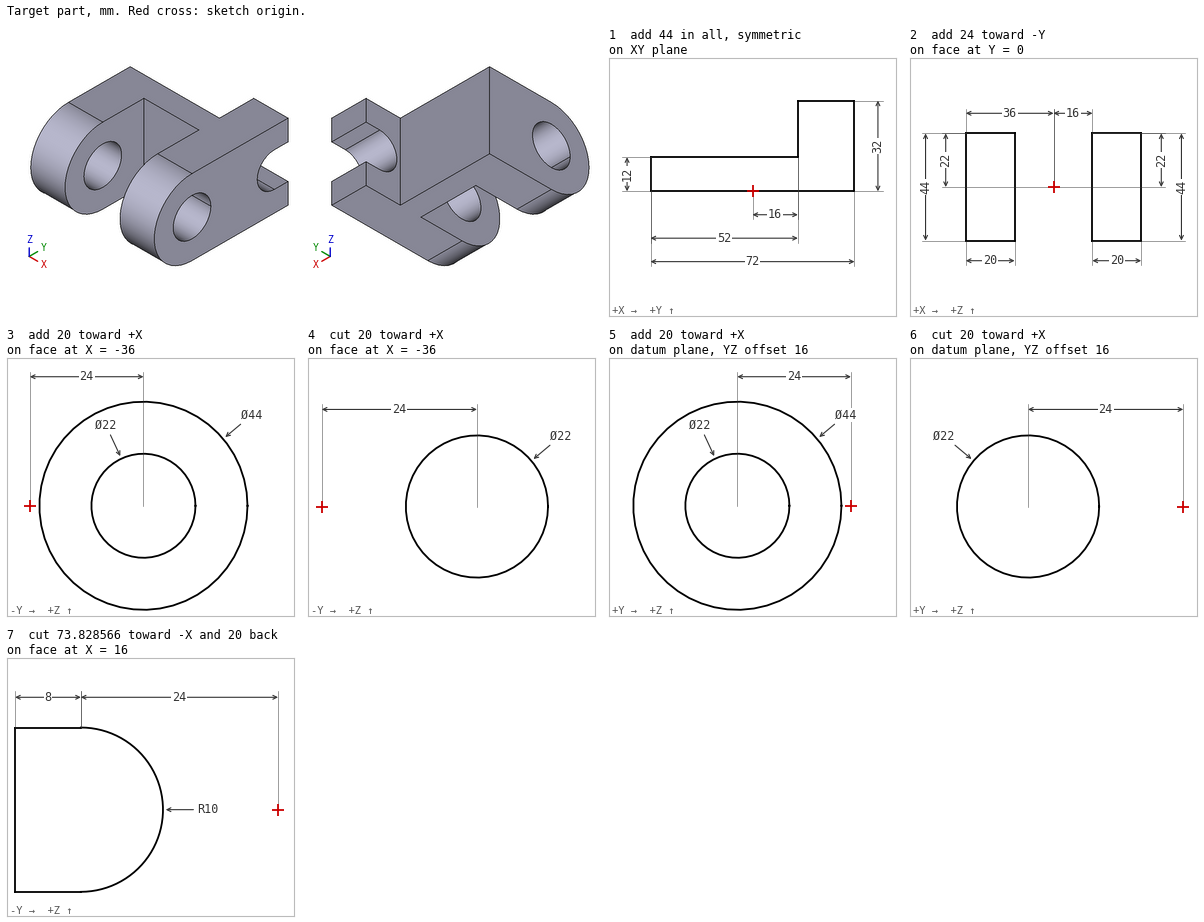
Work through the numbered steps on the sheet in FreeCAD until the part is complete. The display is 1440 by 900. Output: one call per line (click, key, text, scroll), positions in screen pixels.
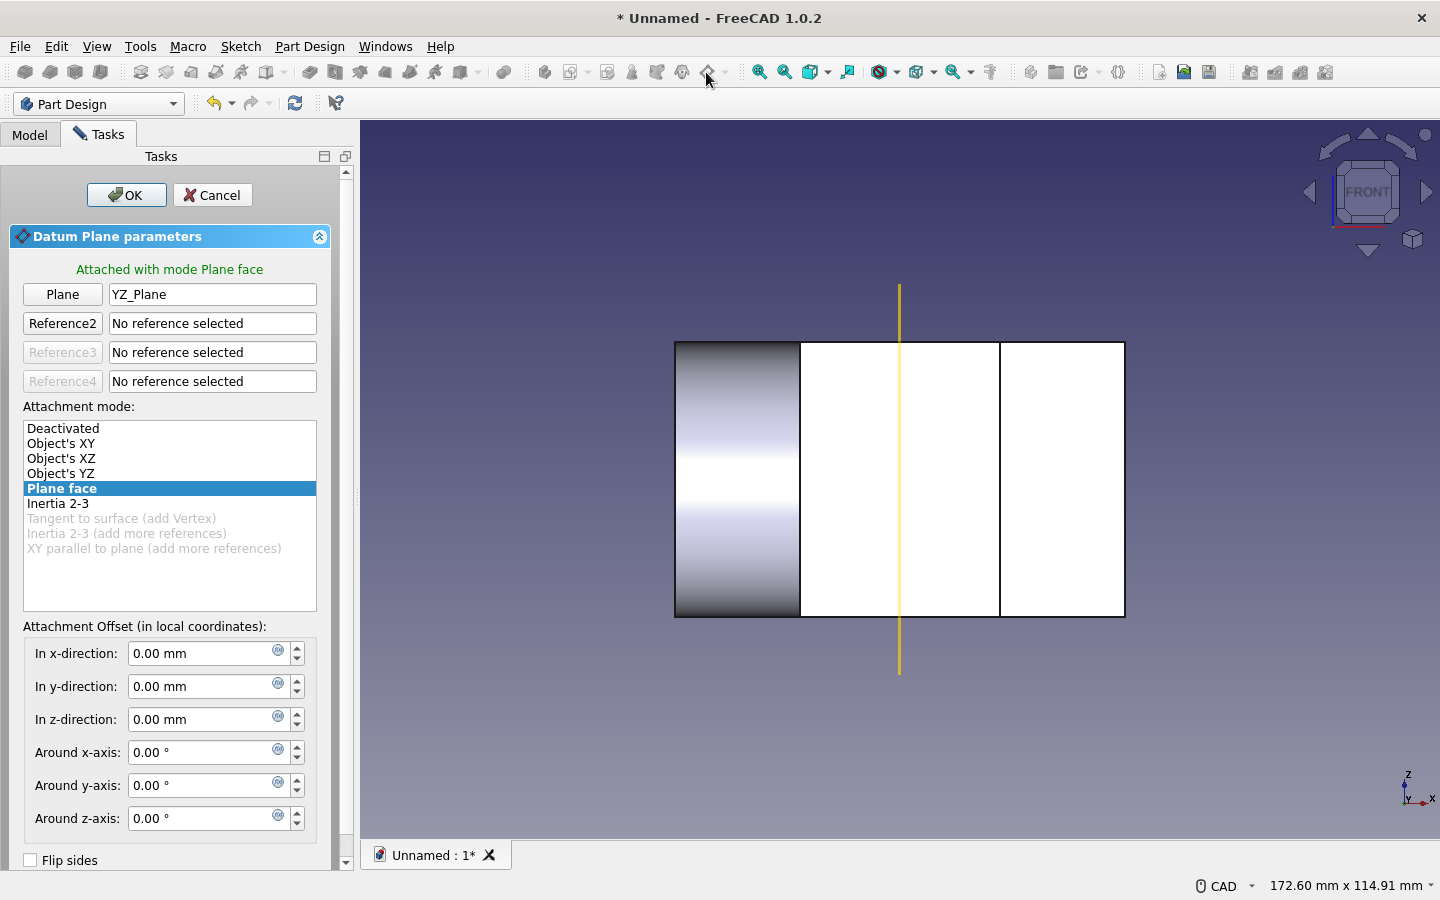
triple_click(210, 720)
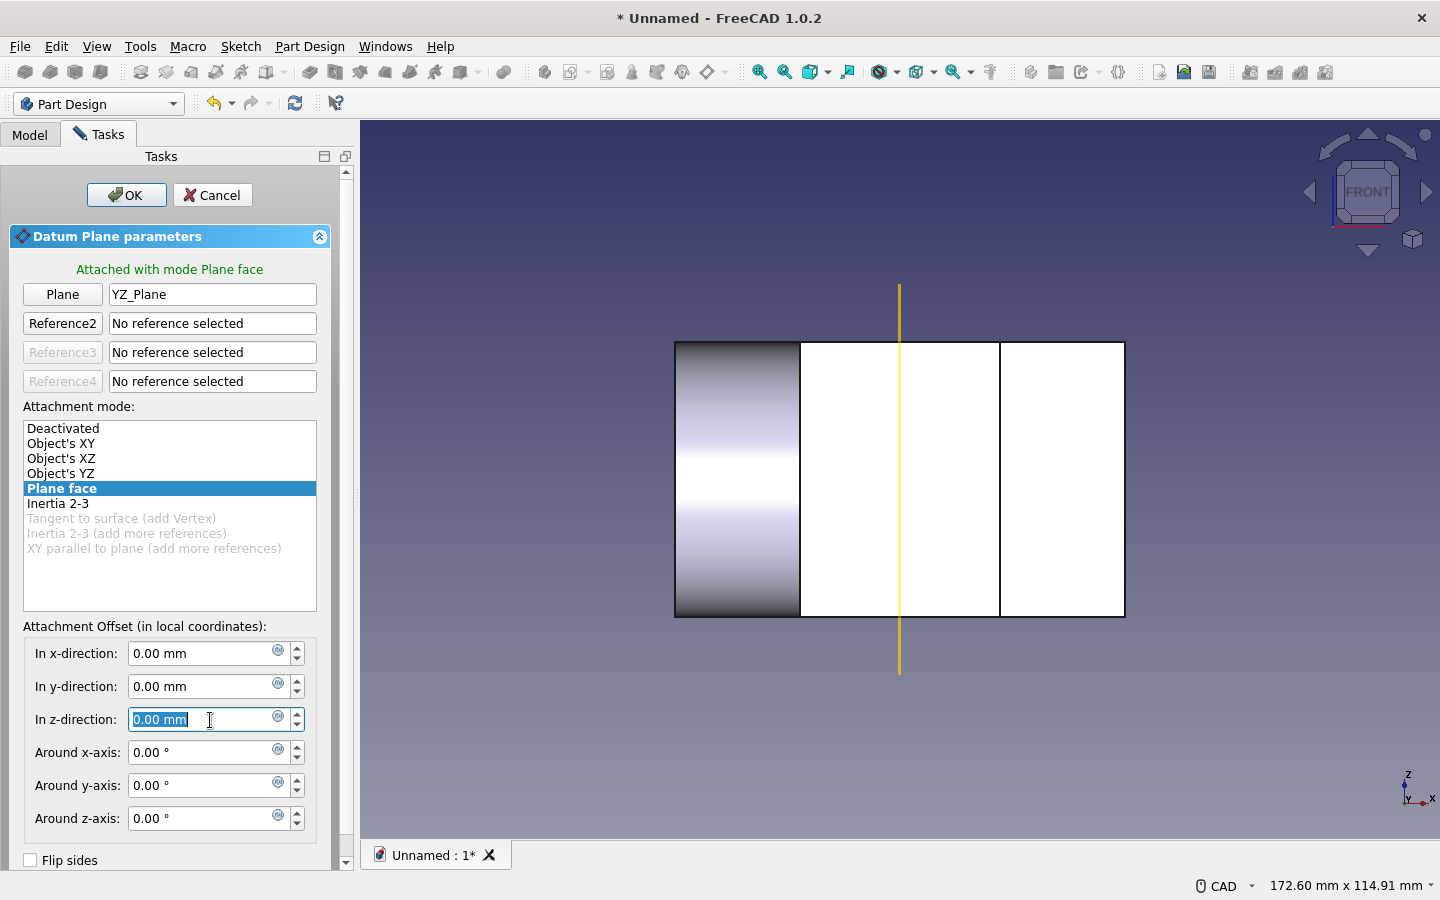
text(16)
key(Tab)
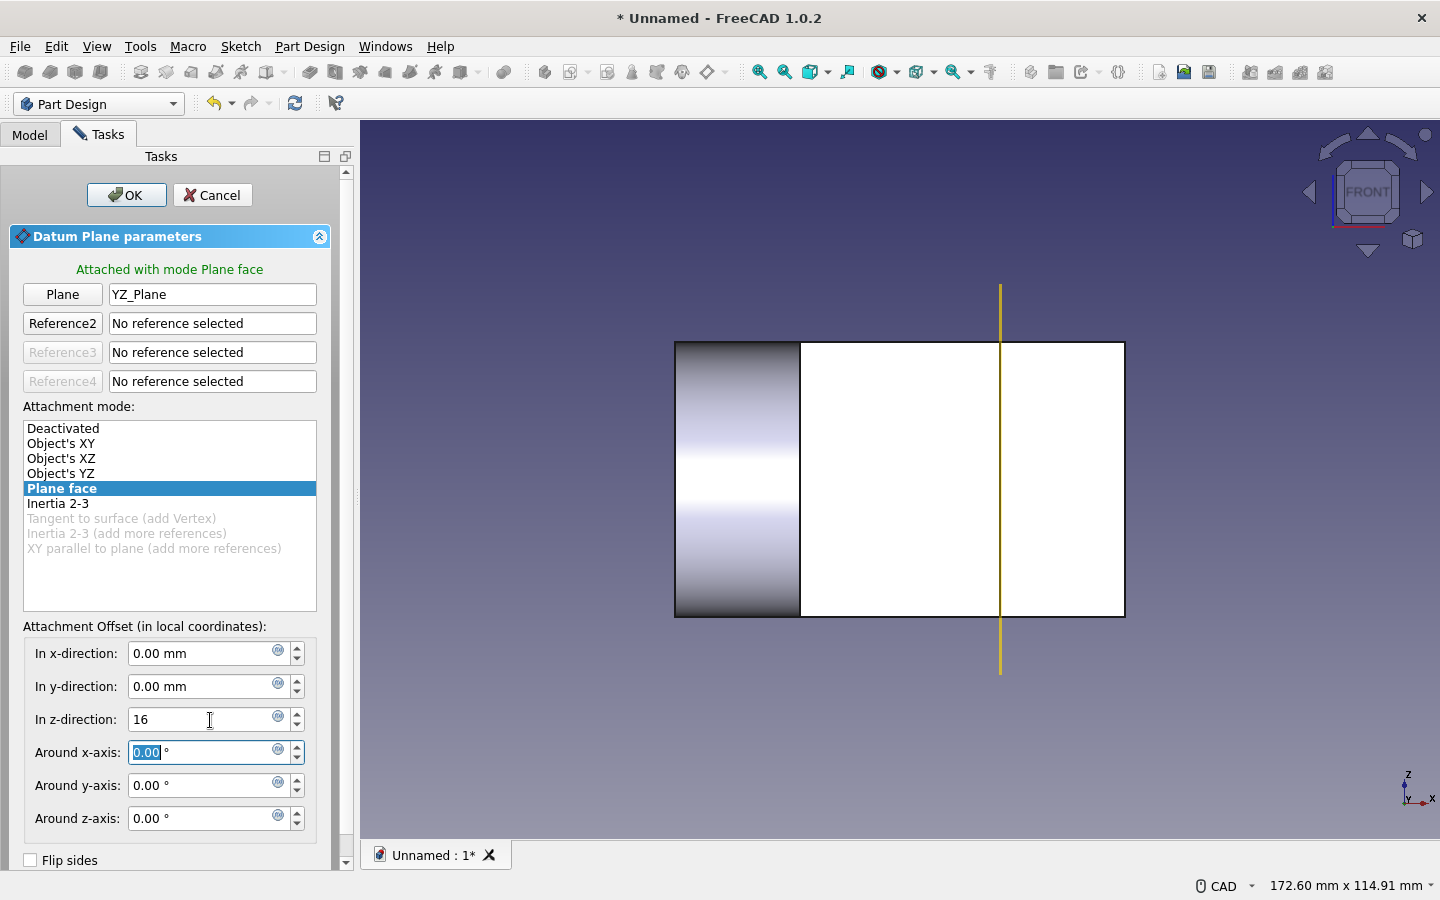
click(127, 195)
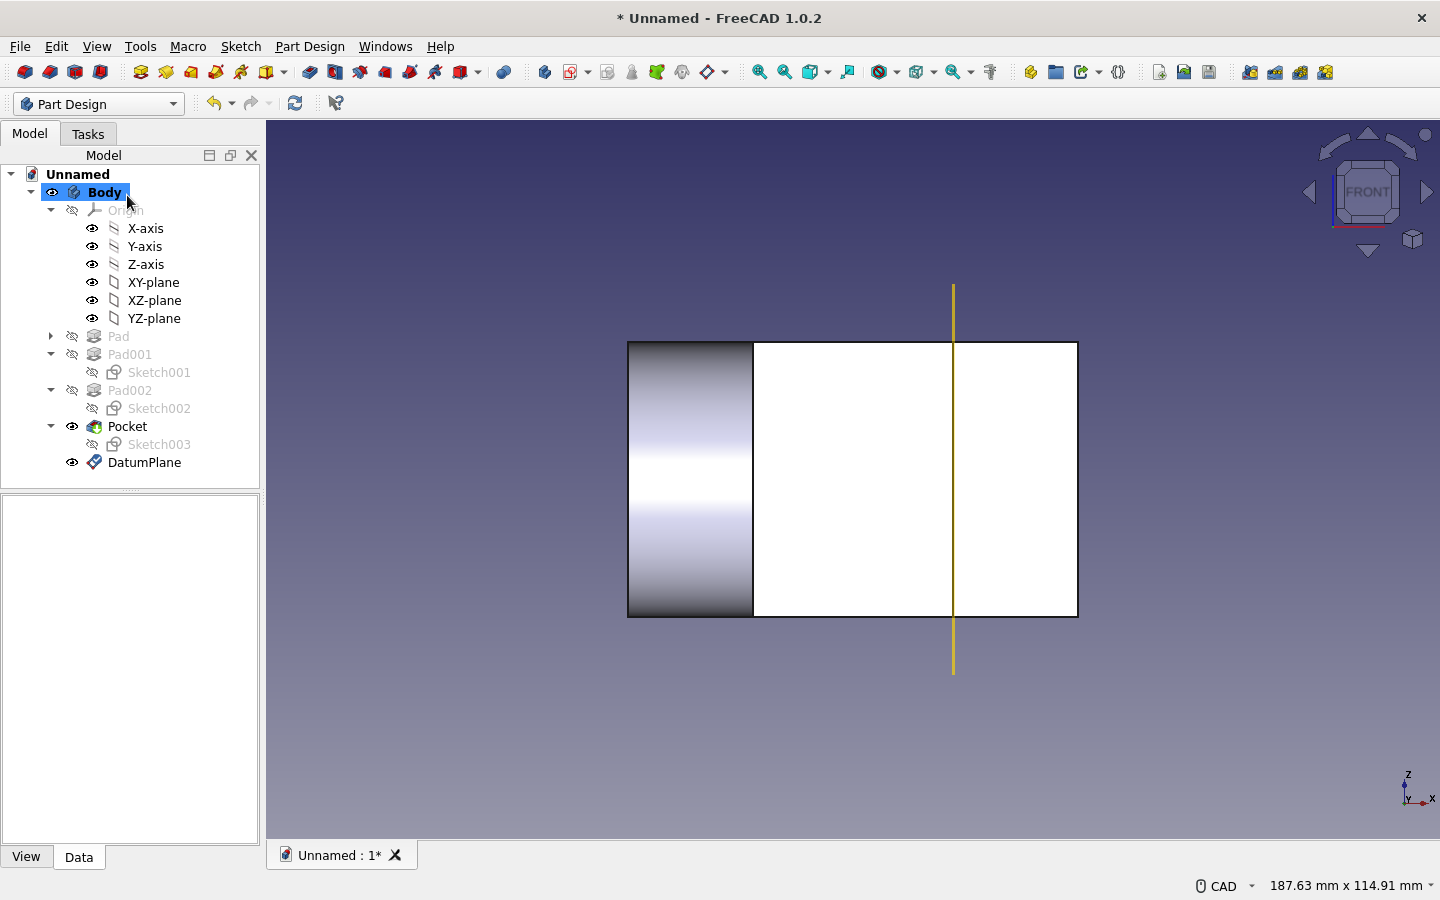
click(117, 462)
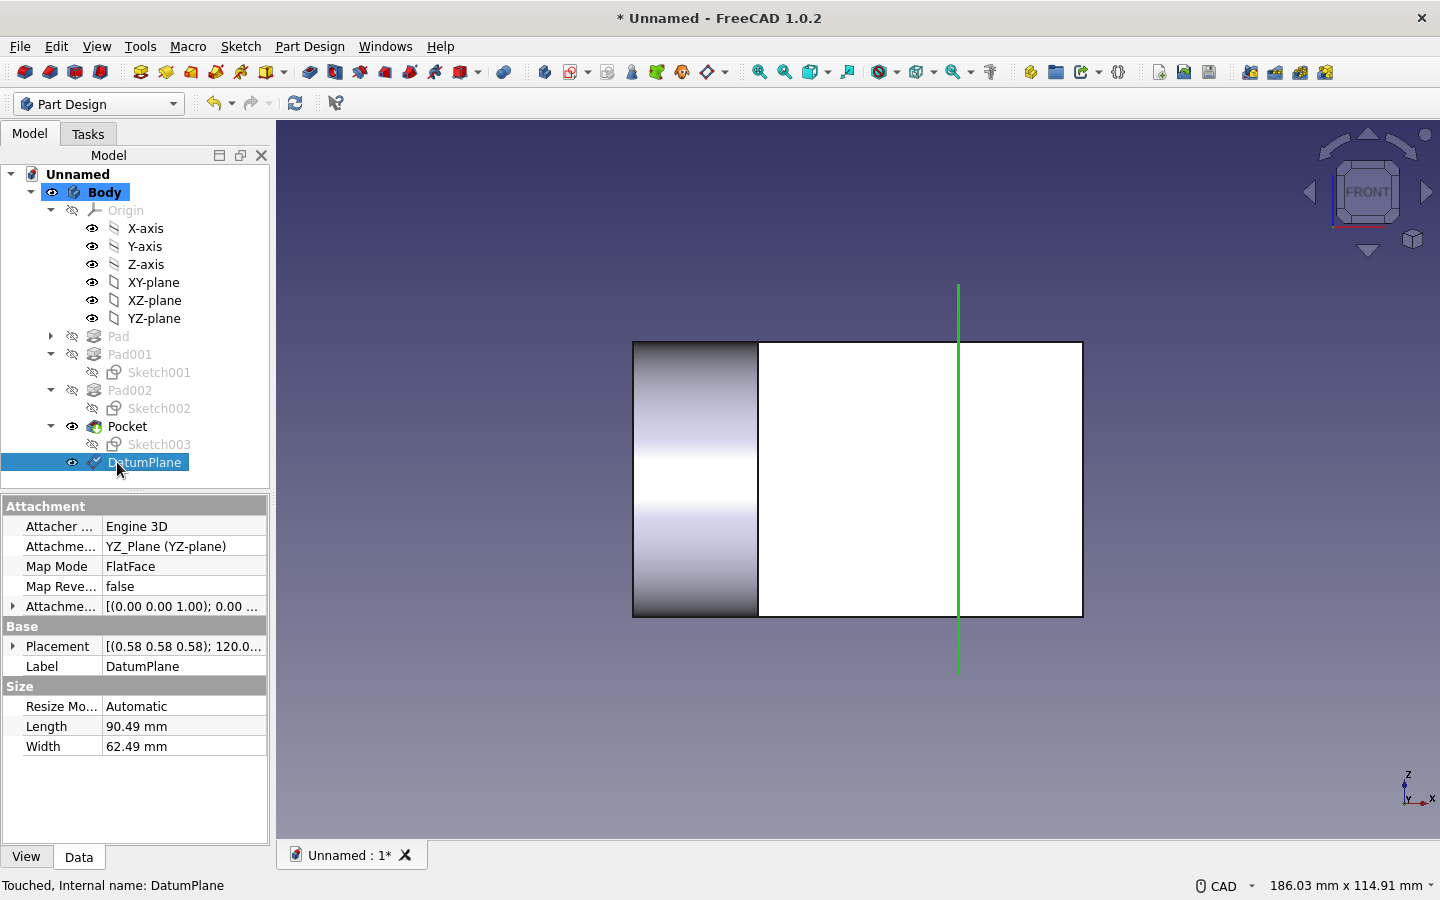
click(570, 72)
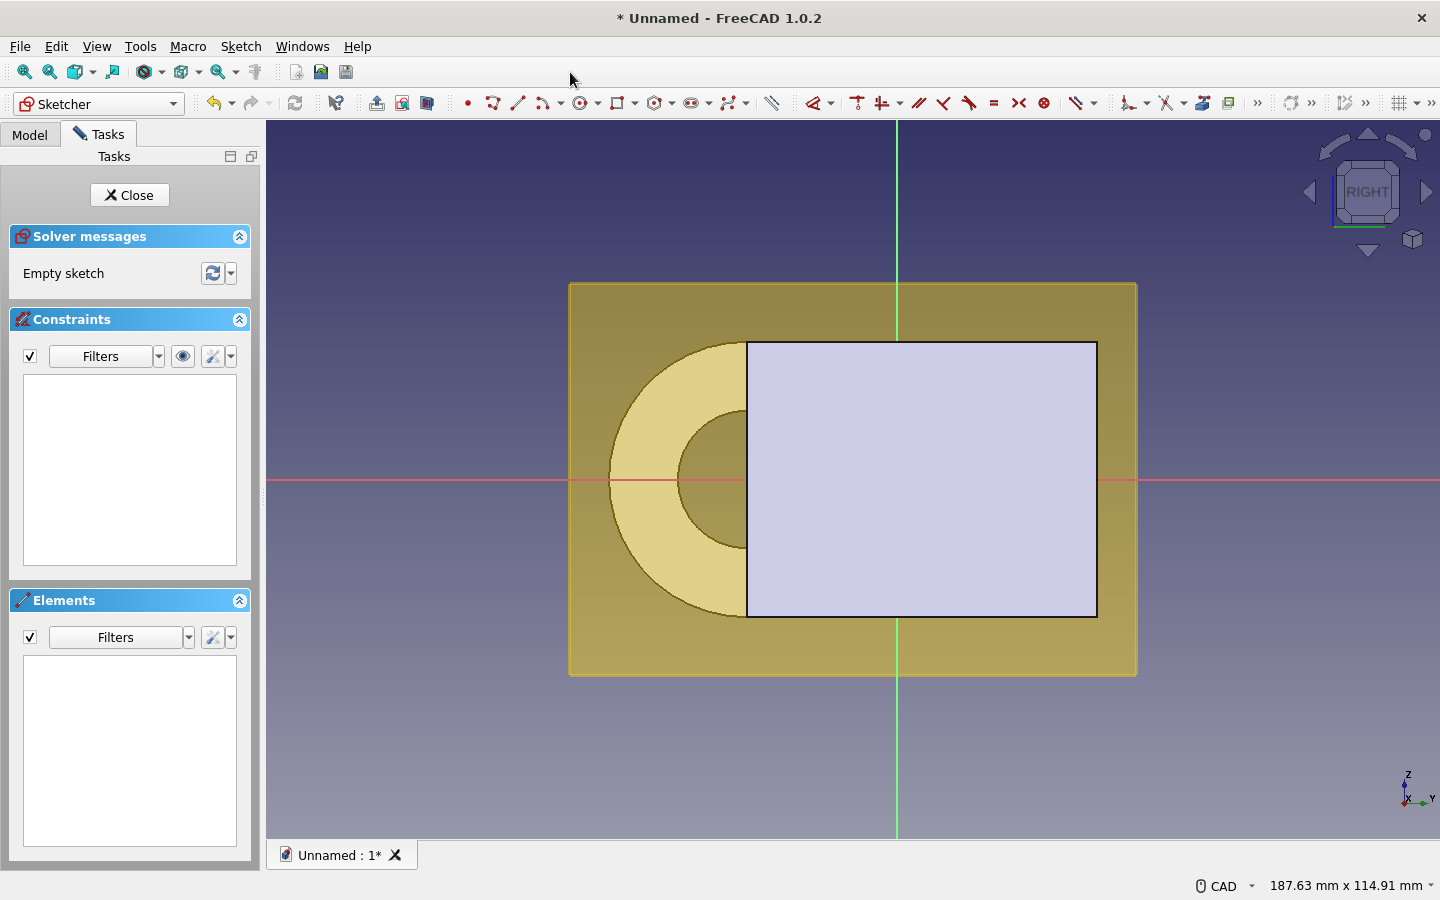
click(427, 104)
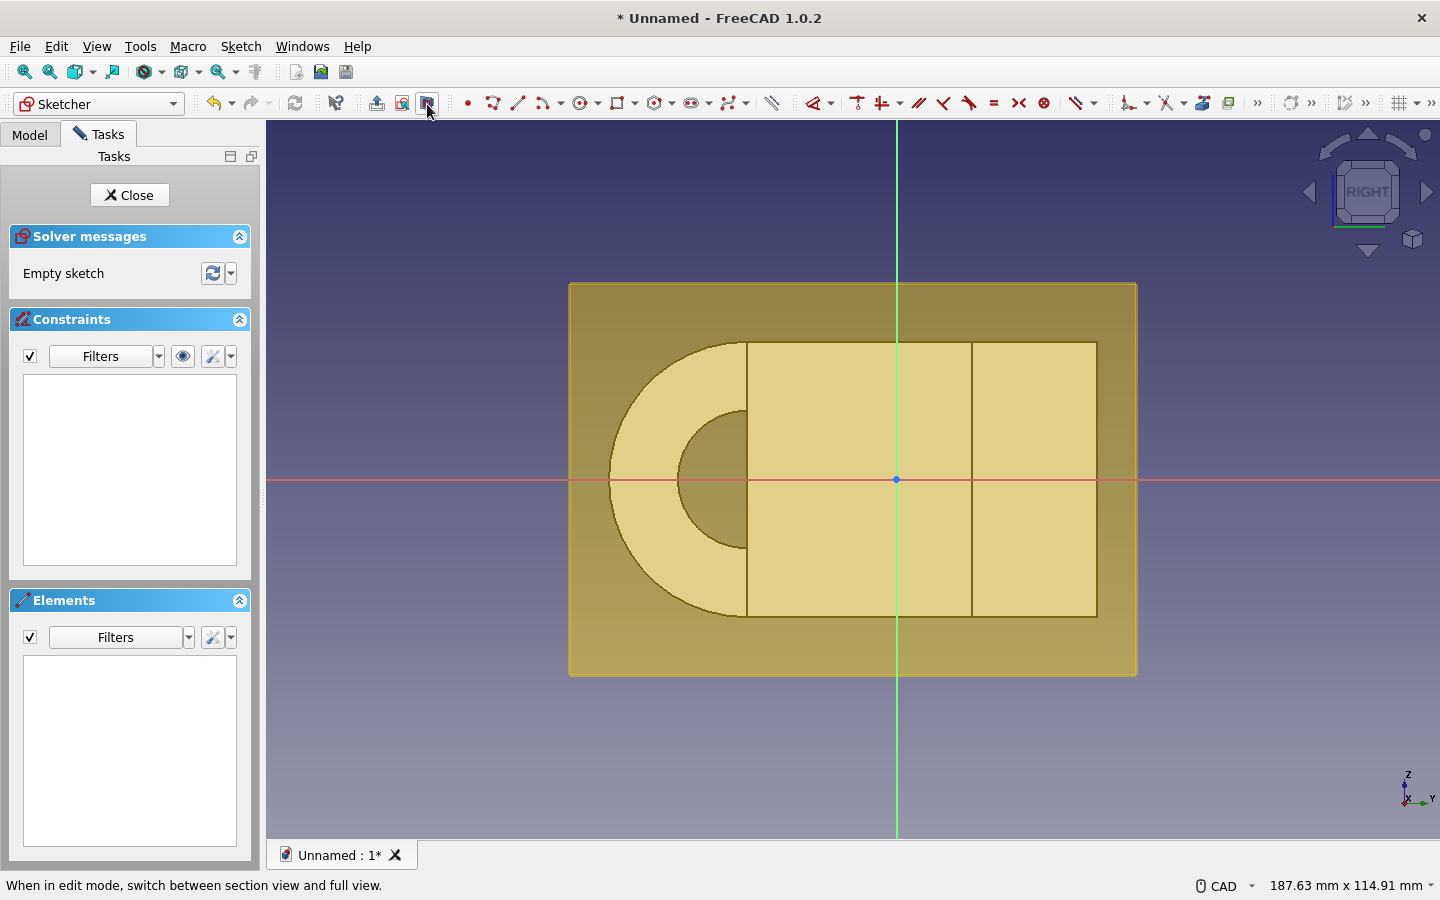
scroll(714, 480, up, 3)